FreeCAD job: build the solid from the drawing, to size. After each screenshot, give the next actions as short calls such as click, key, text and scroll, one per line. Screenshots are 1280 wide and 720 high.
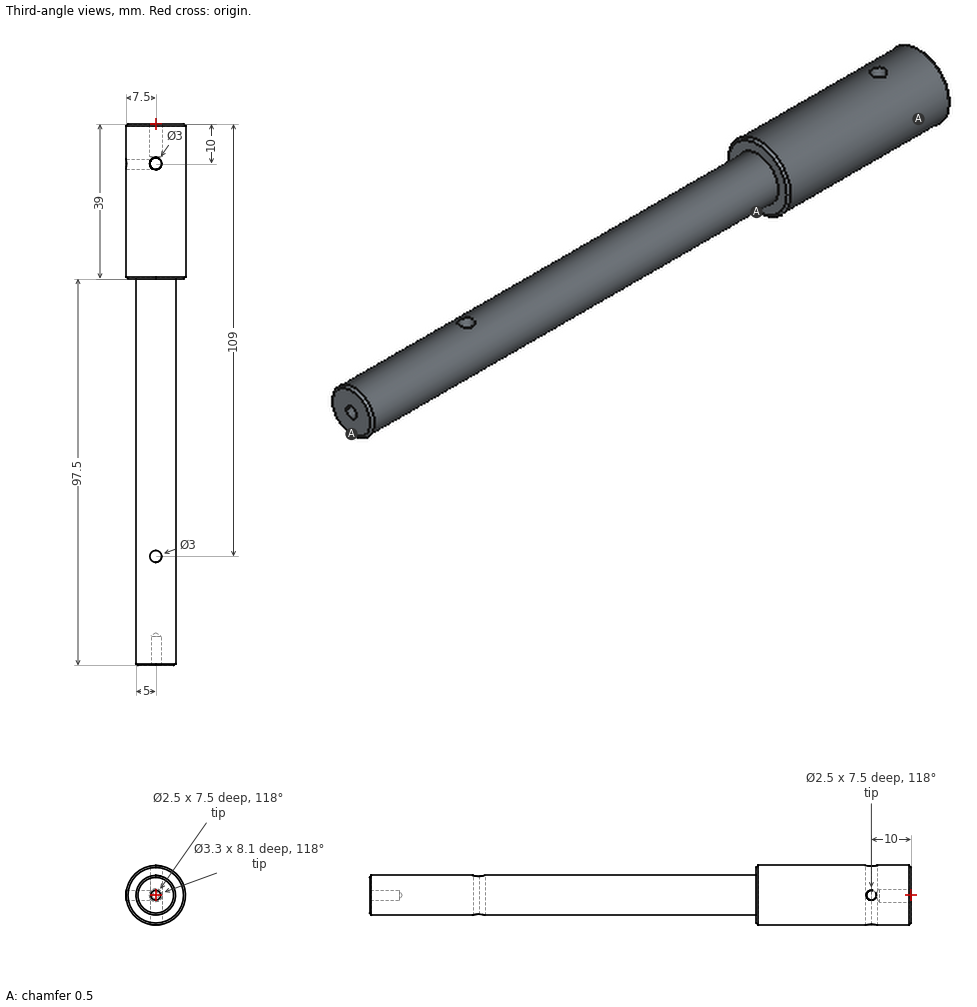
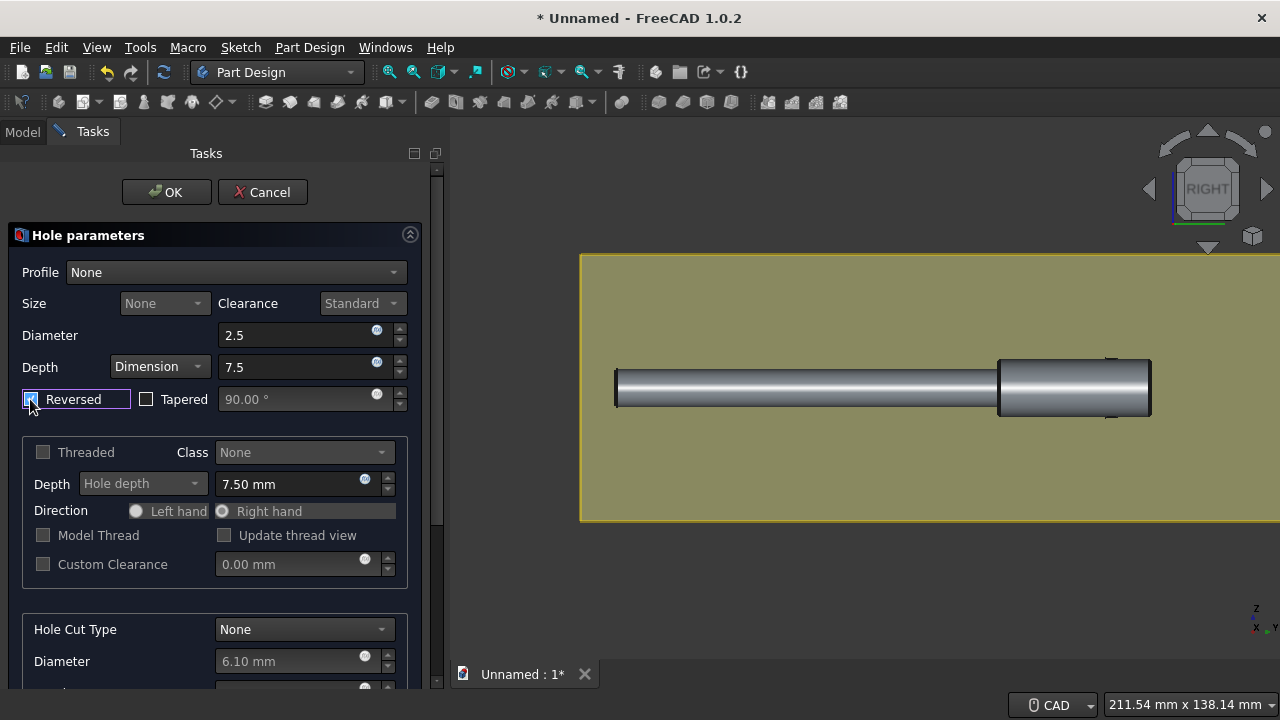
click(167, 192)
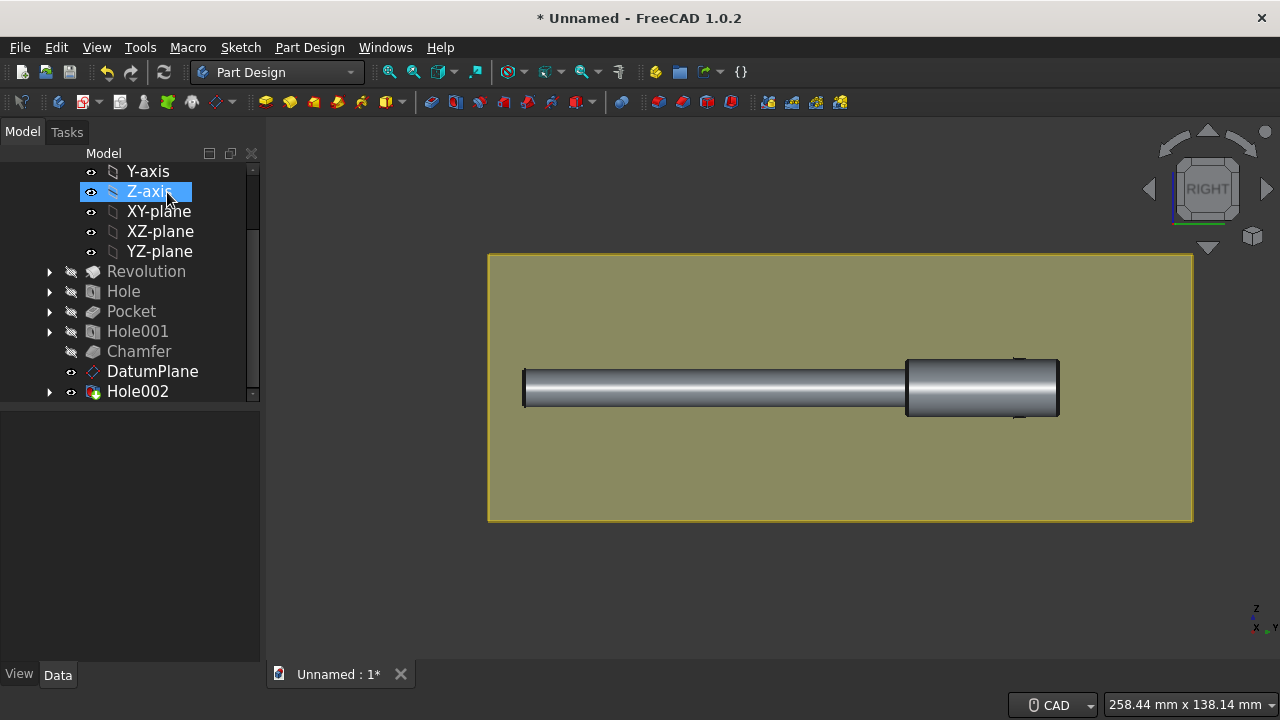
click(116, 372)
key(space)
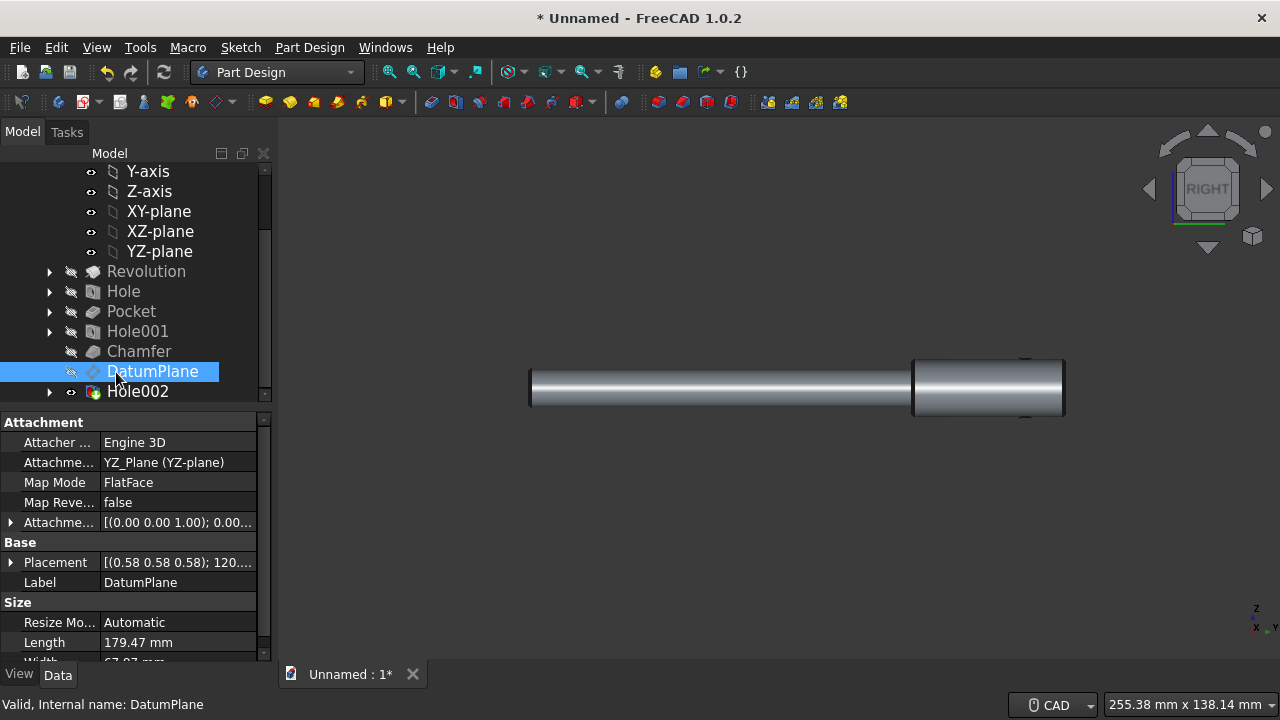
click(318, 619)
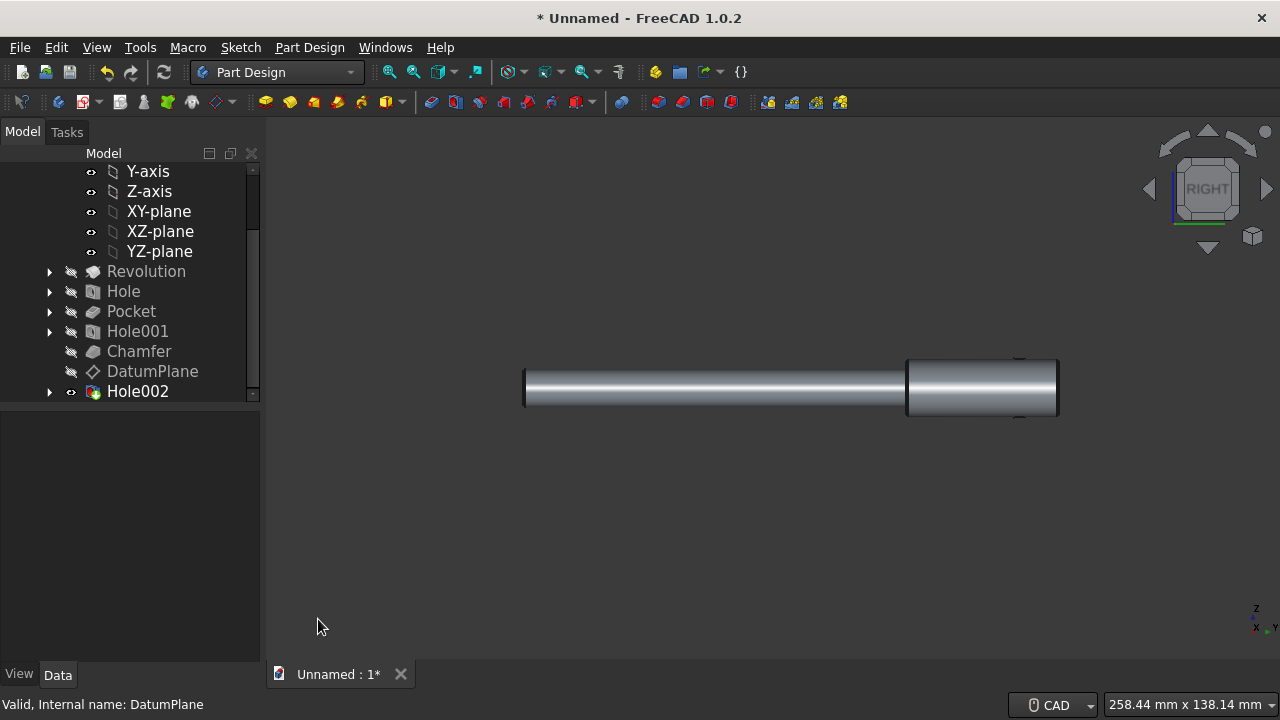
click(84, 102)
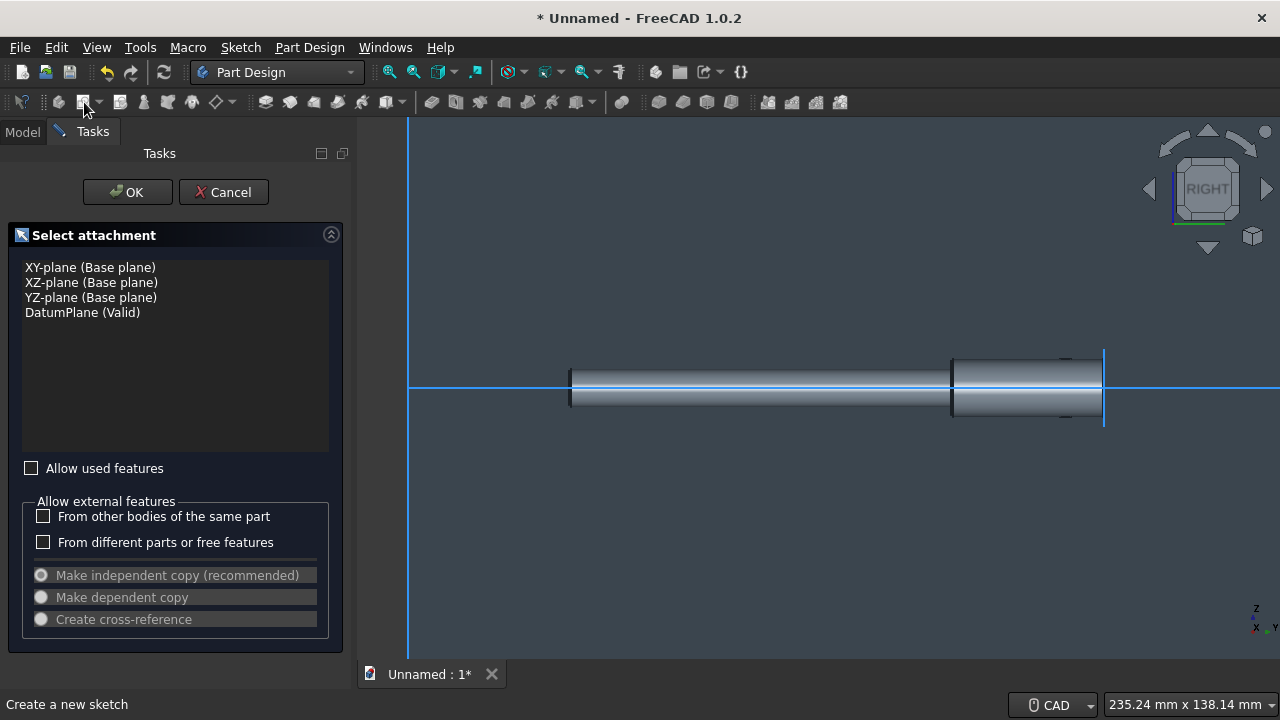
click(82, 268)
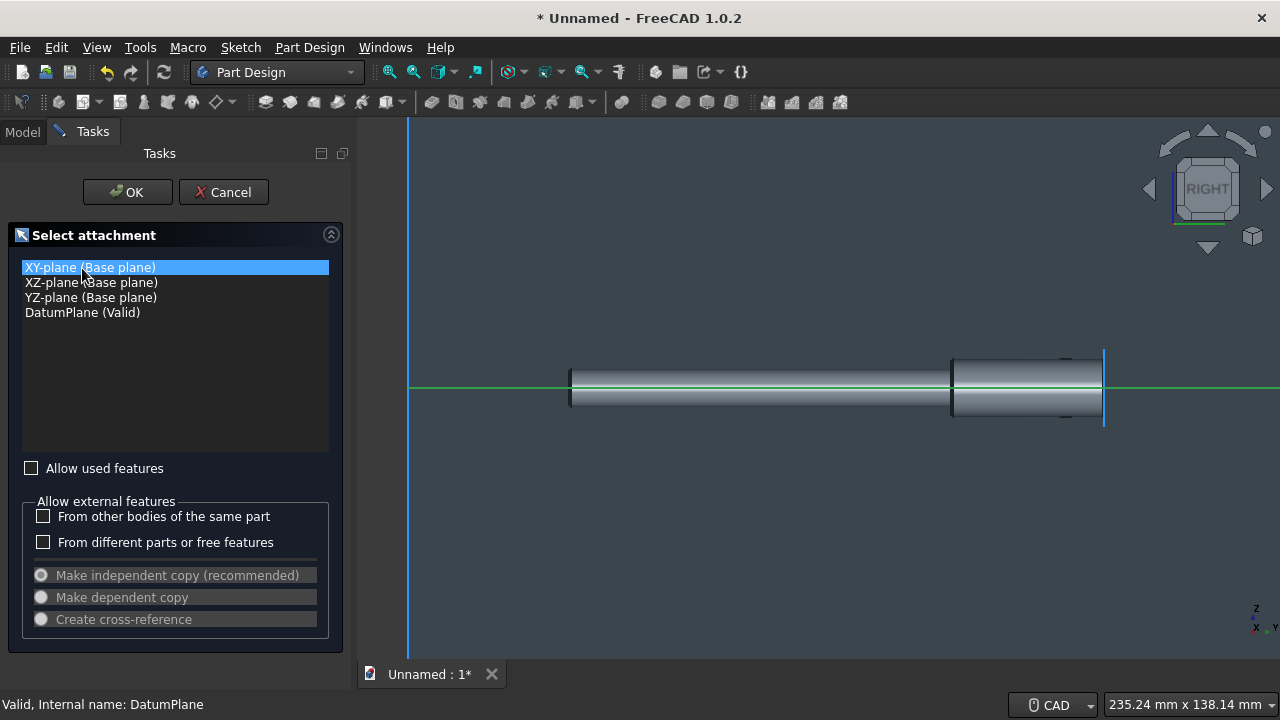
click(128, 192)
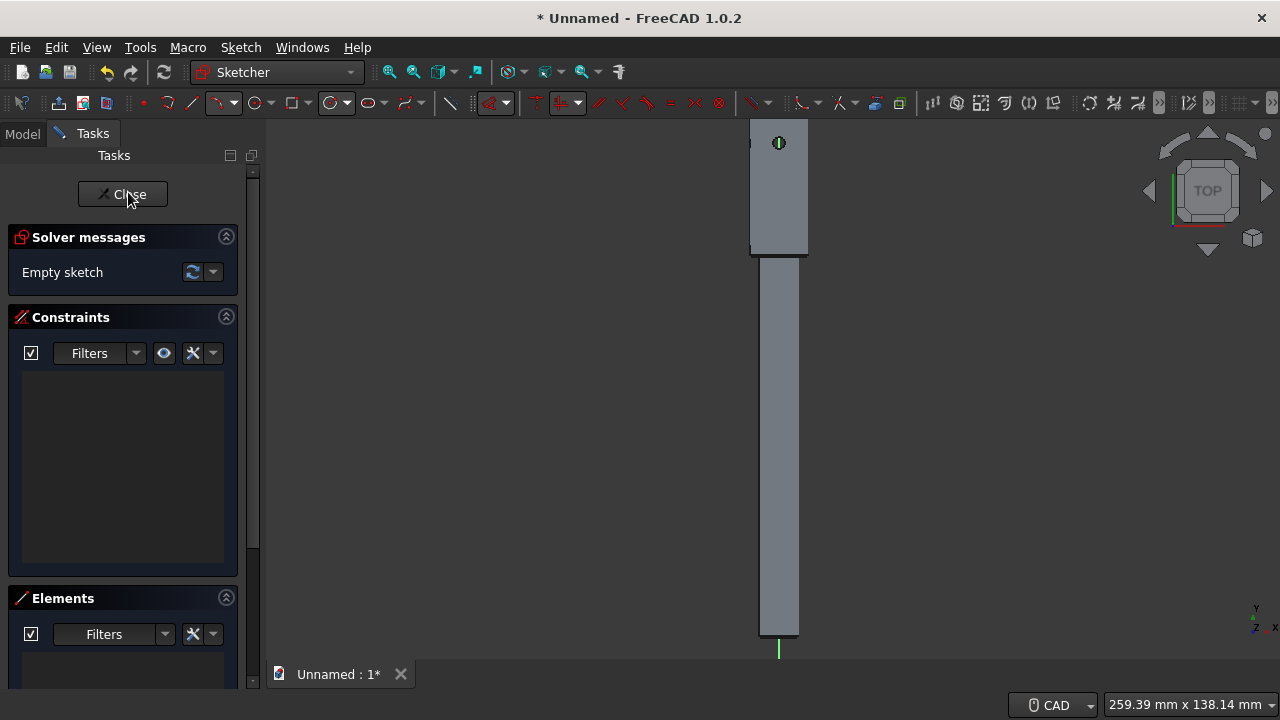
click(108, 104)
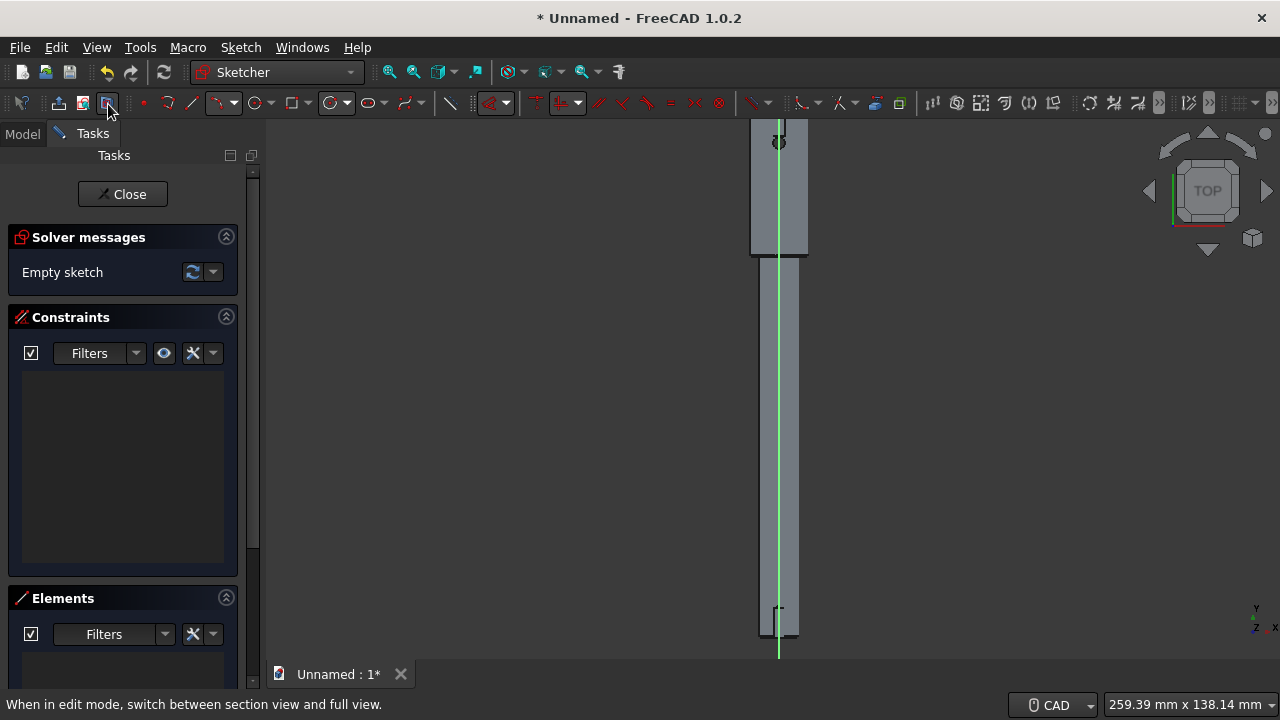
scroll(783, 538, up, 15)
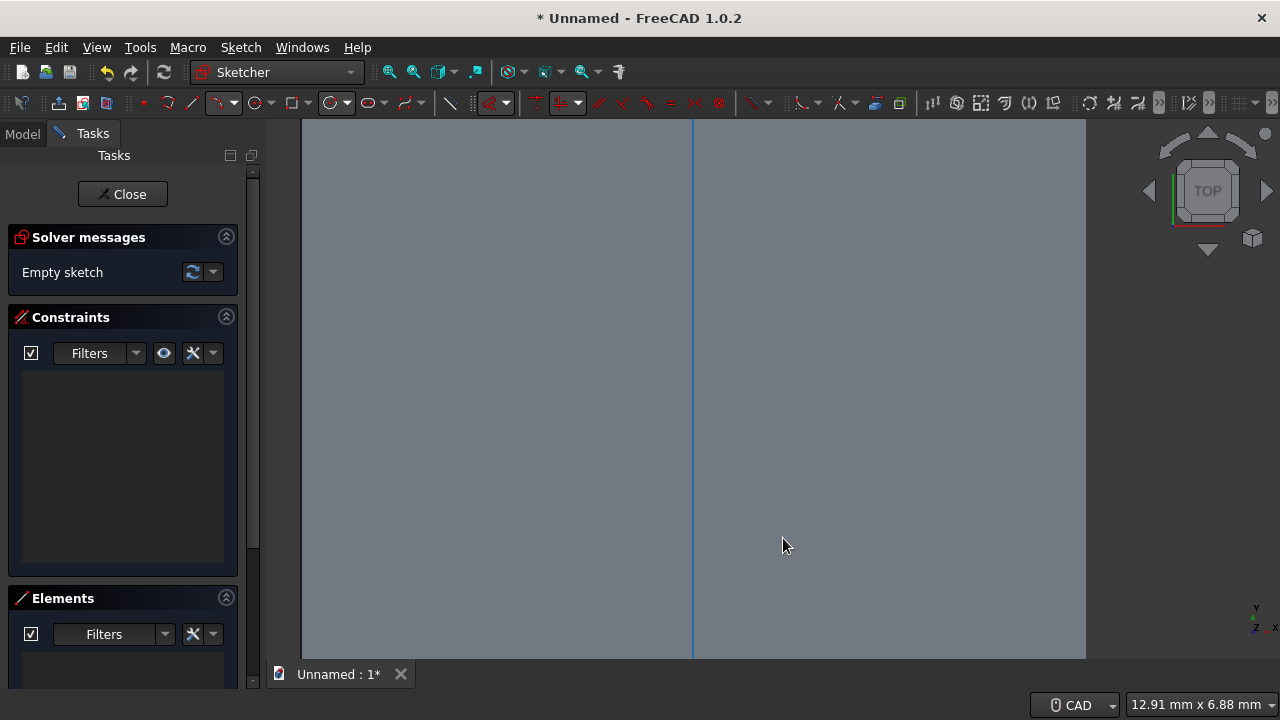
scroll(670, 318, up, 2)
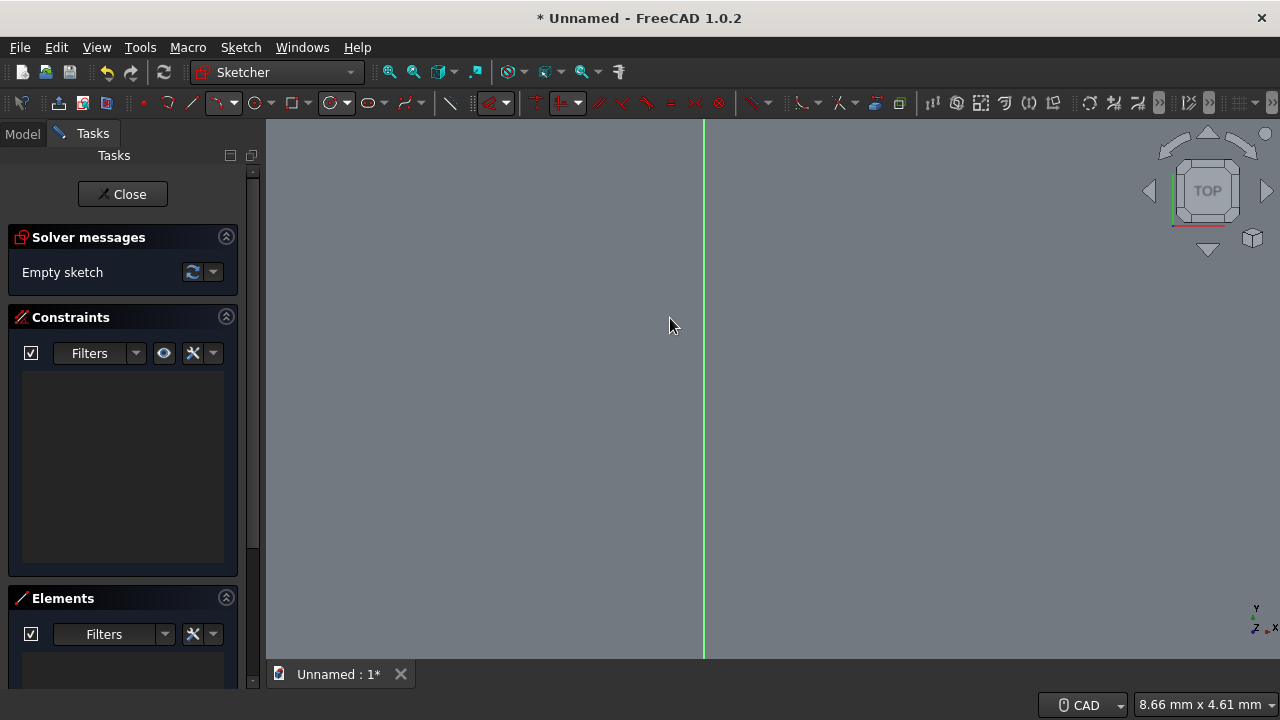
click(256, 104)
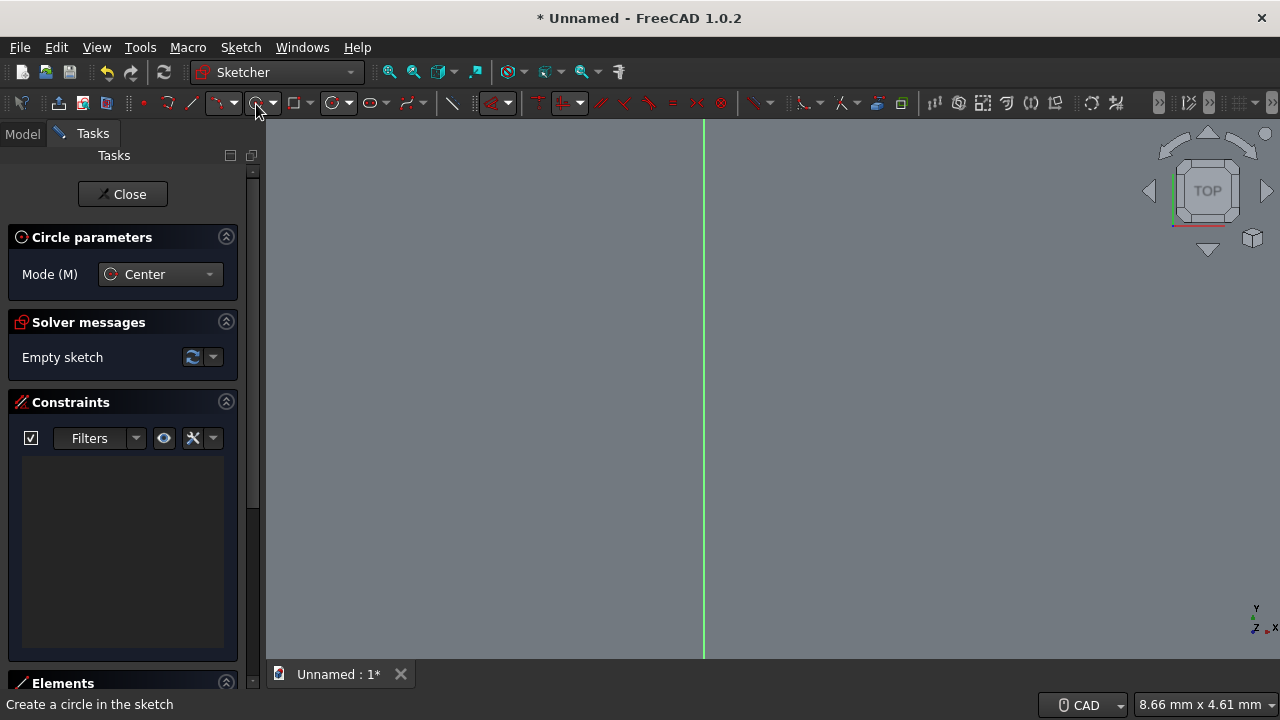
click(704, 389)
click(829, 265)
key(Escape)